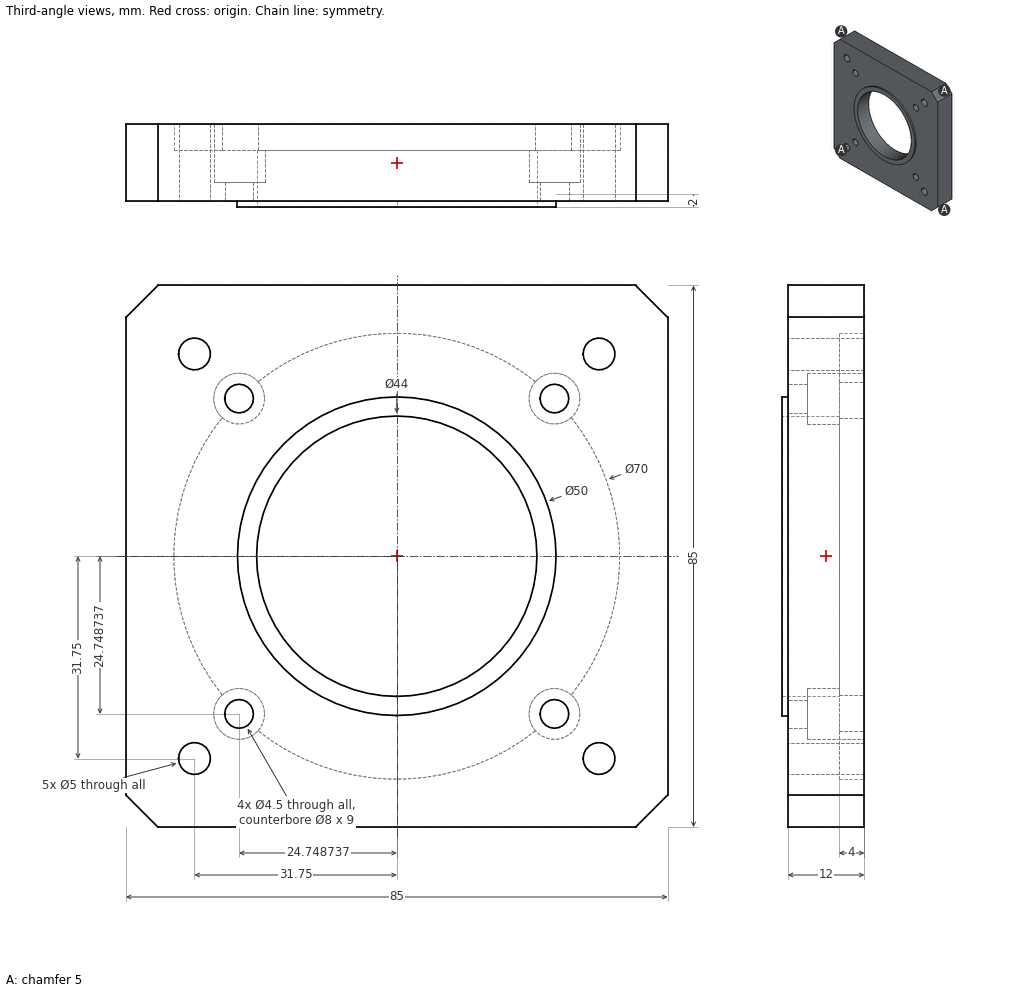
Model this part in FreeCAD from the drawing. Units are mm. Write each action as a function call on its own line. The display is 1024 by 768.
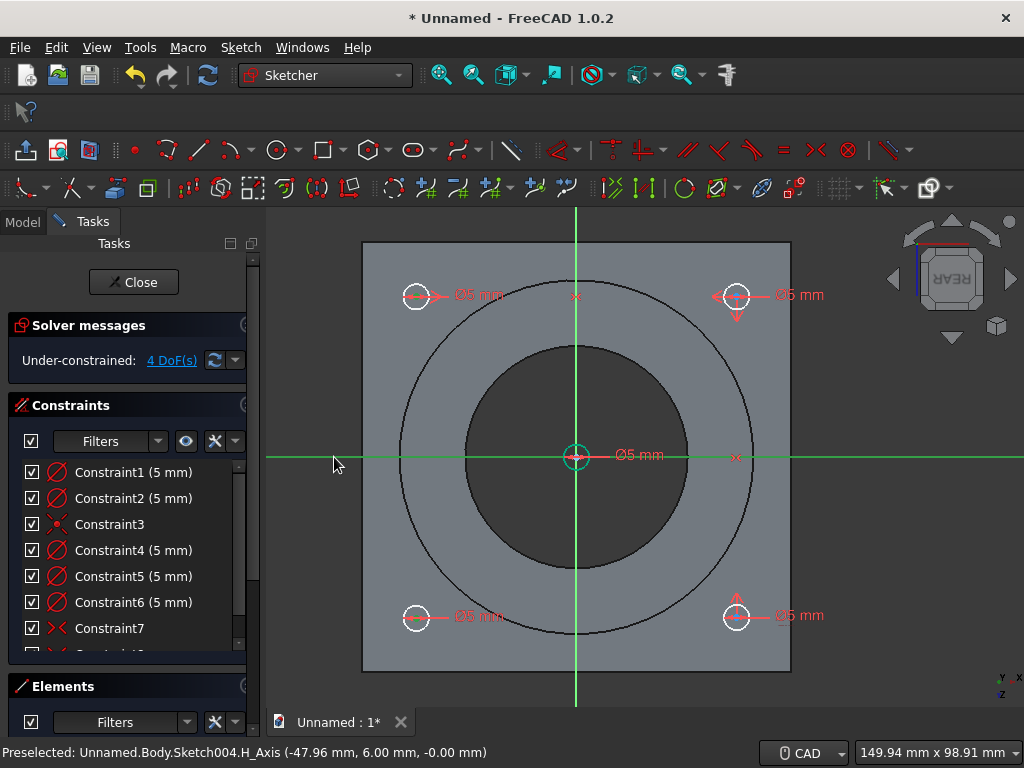
click(816, 150)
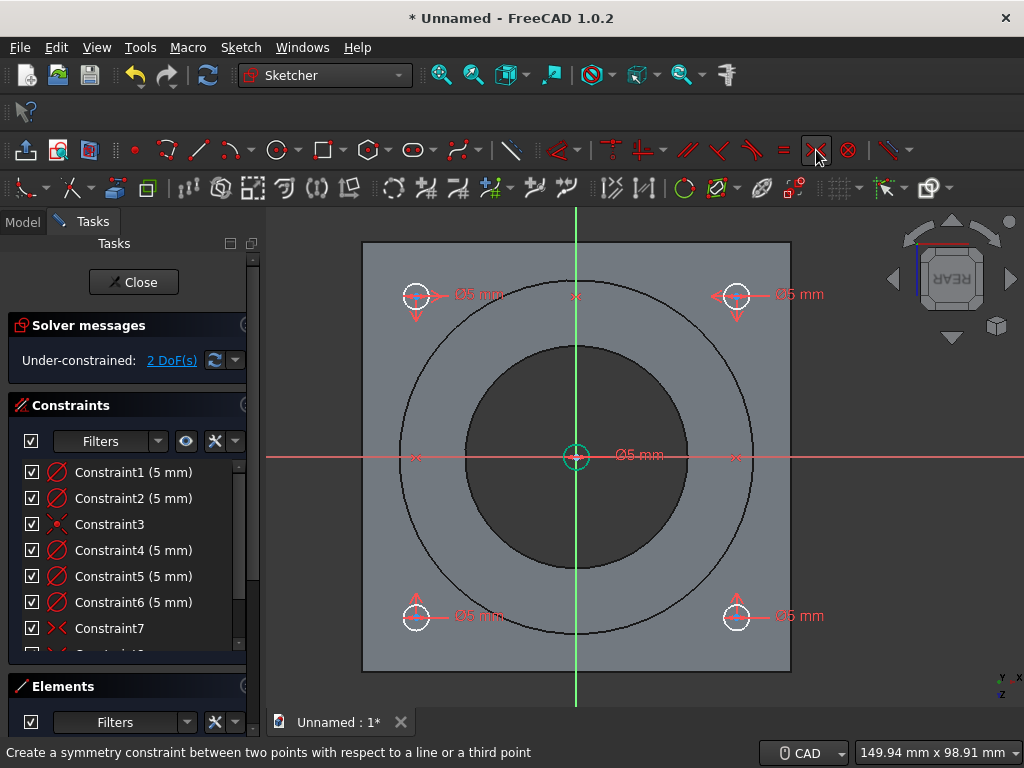
key(d)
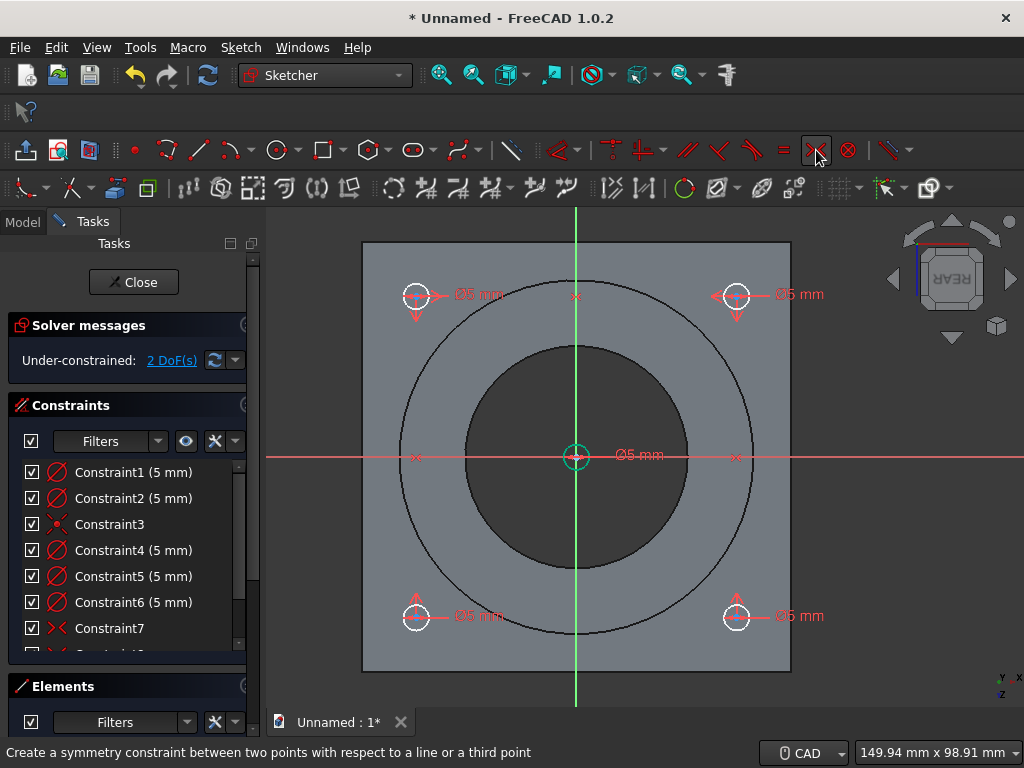
click(416, 296)
click(496, 262)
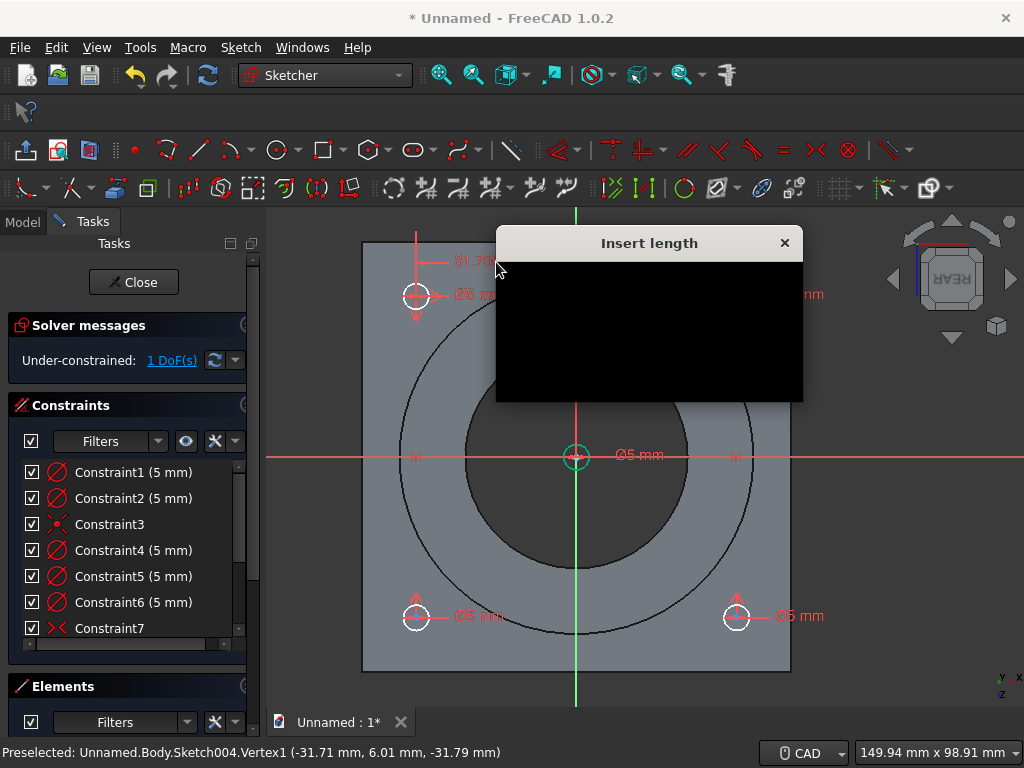
text(31.75)
key(Return)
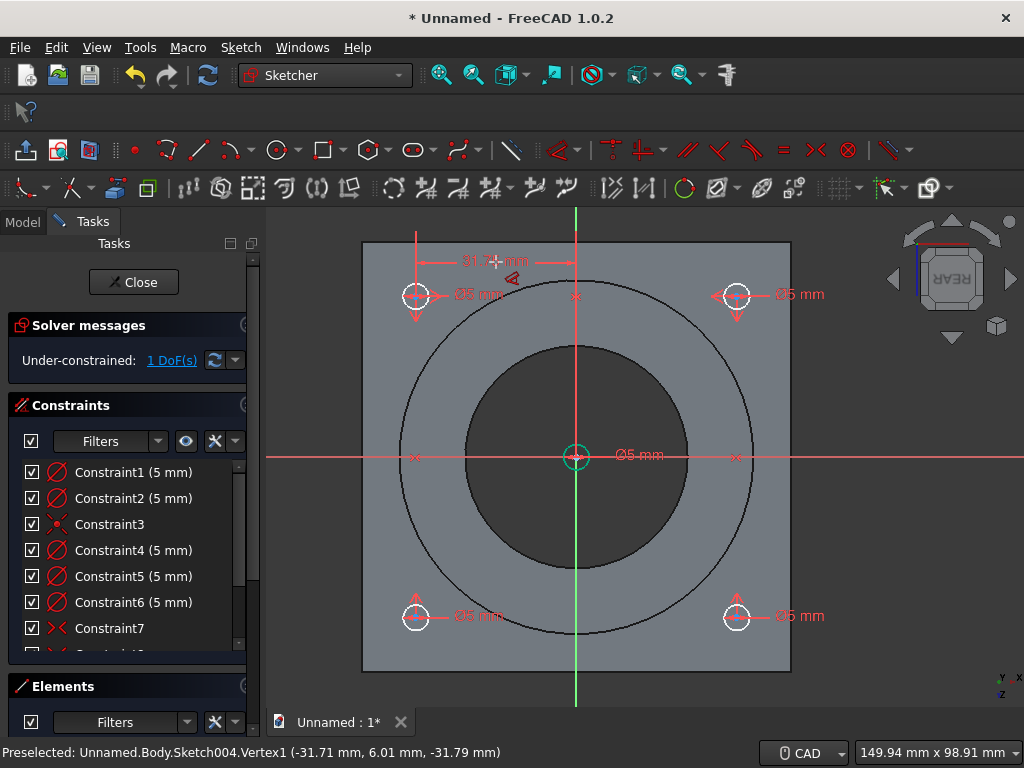
click(416, 296)
click(382, 377)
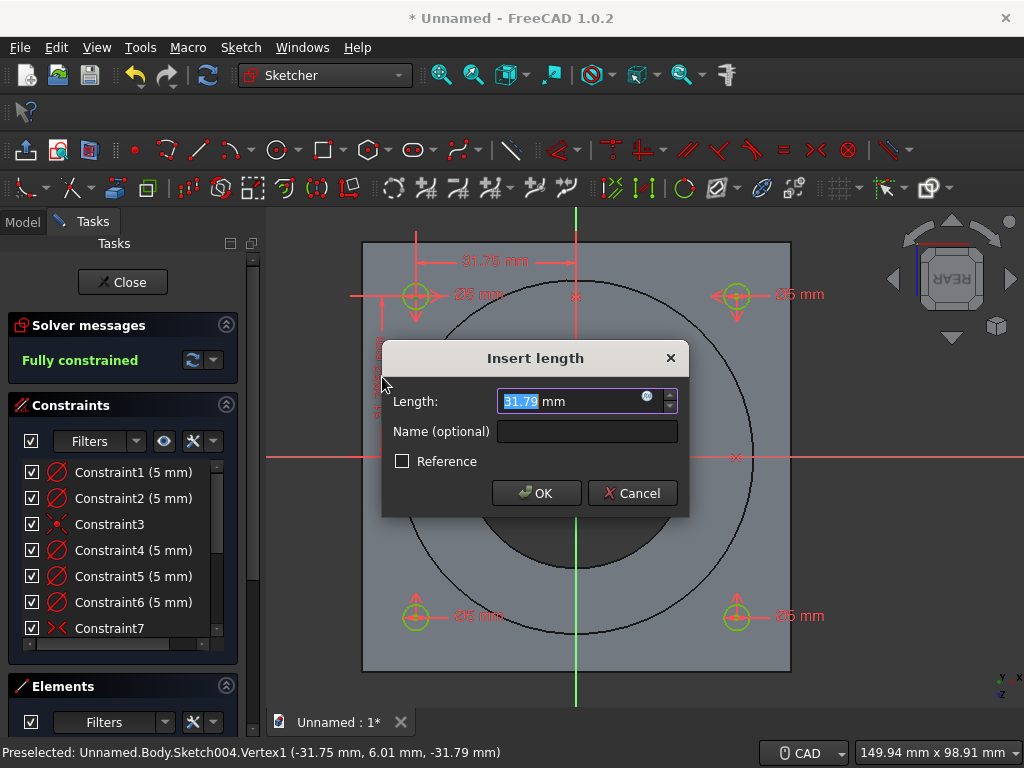
text(31.75)
key(Return)
key(Escape)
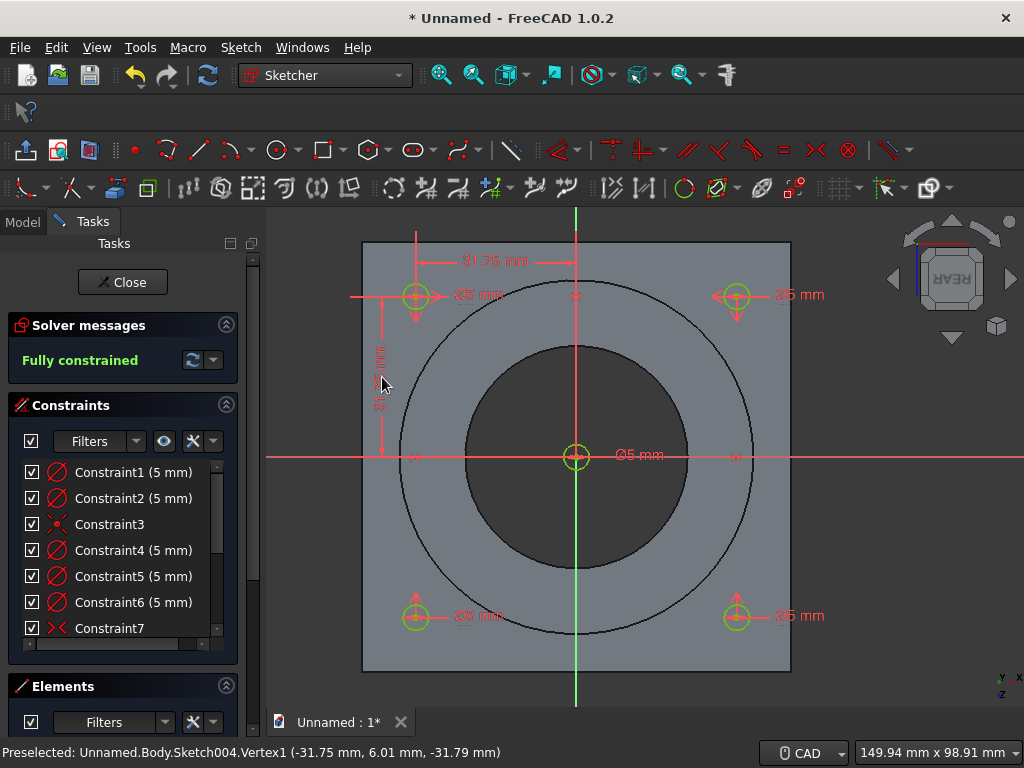
click(123, 282)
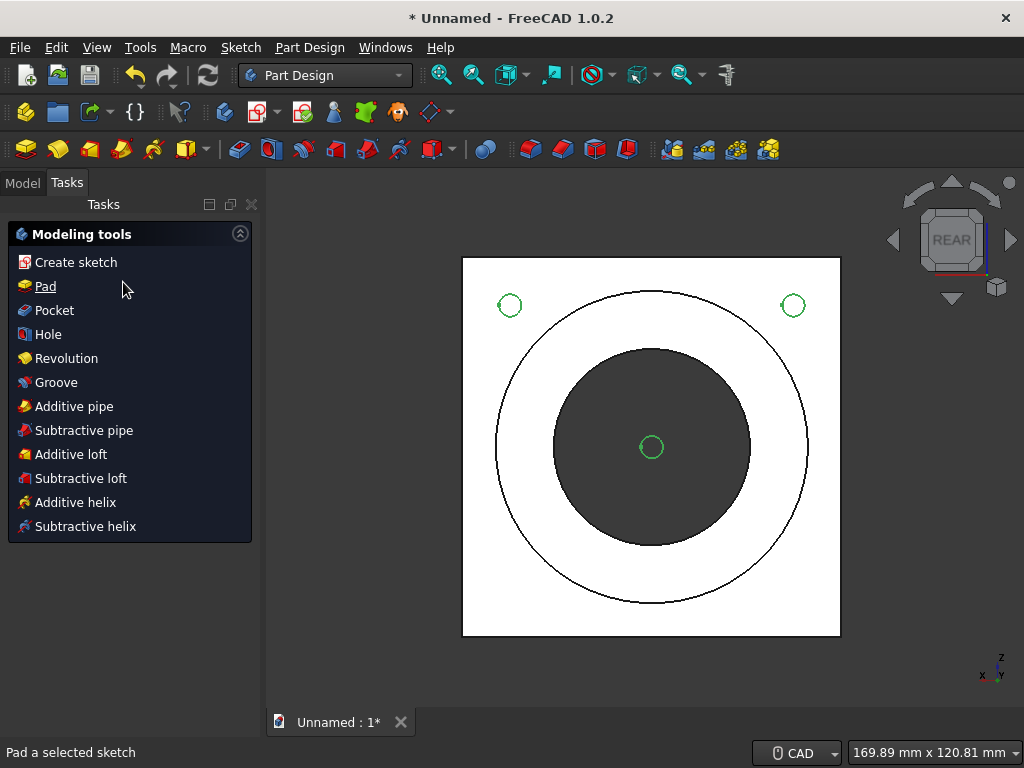
click(272, 150)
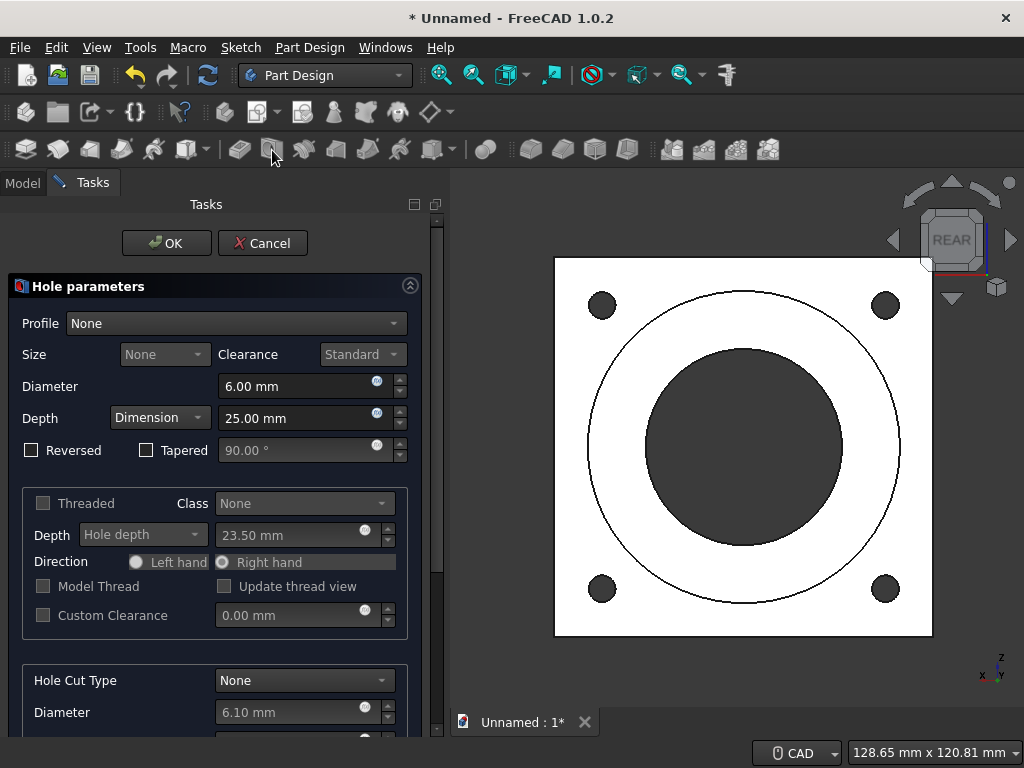
triple_click(305, 386)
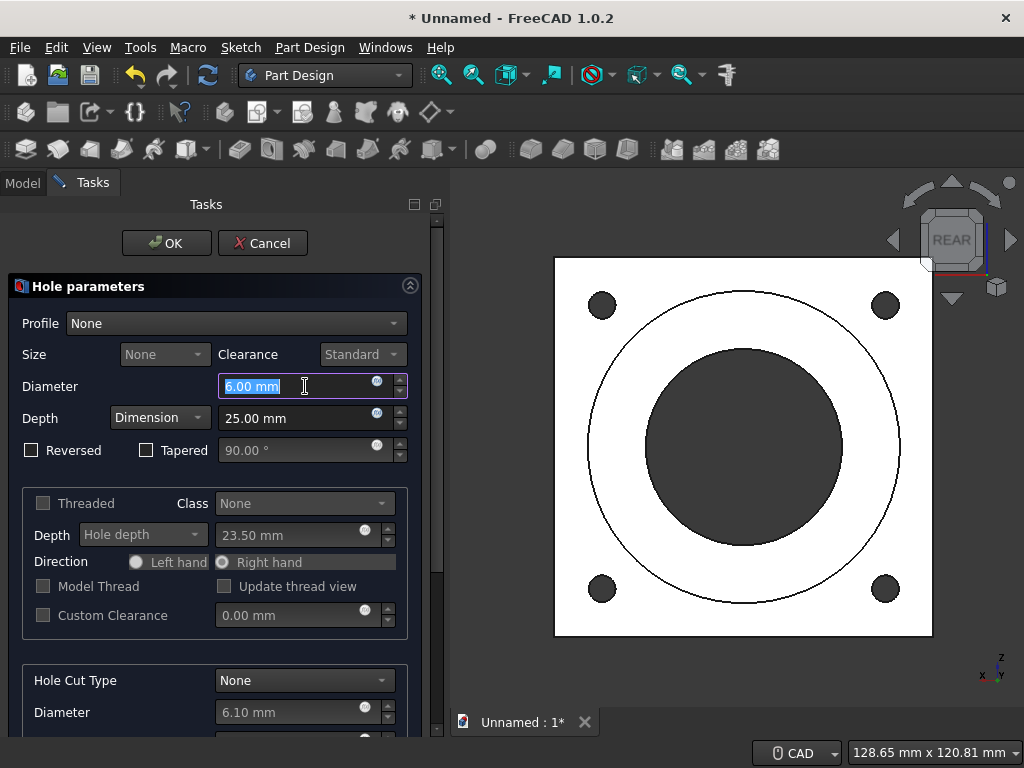
text(5)
key(Tab)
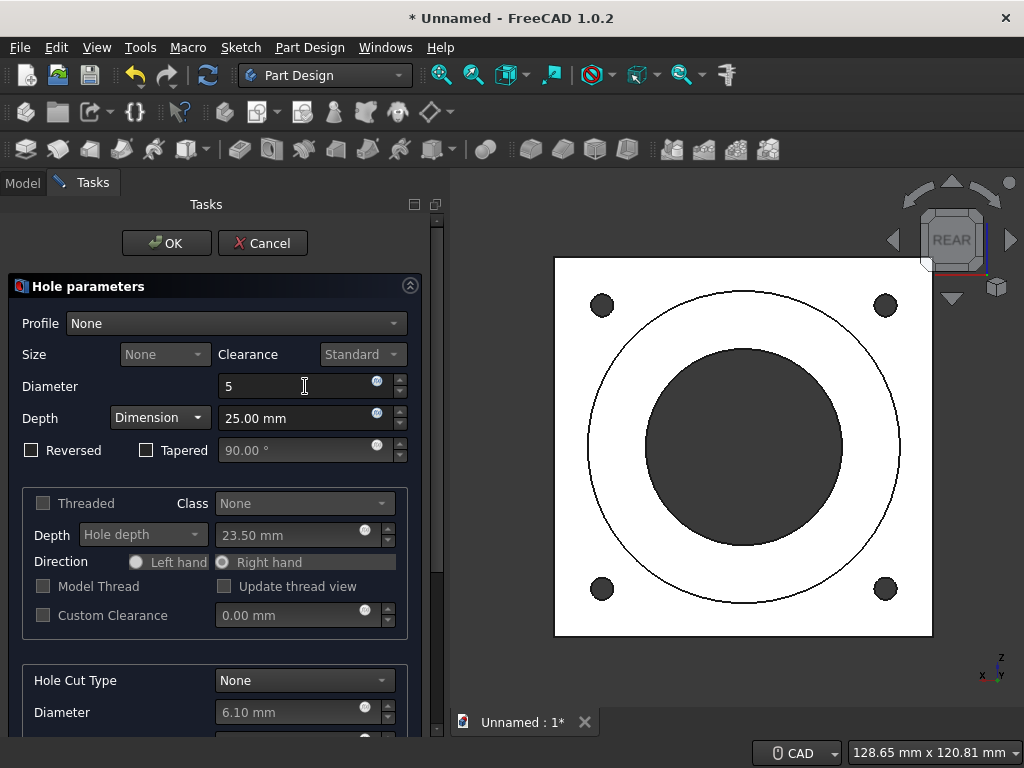
click(161, 418)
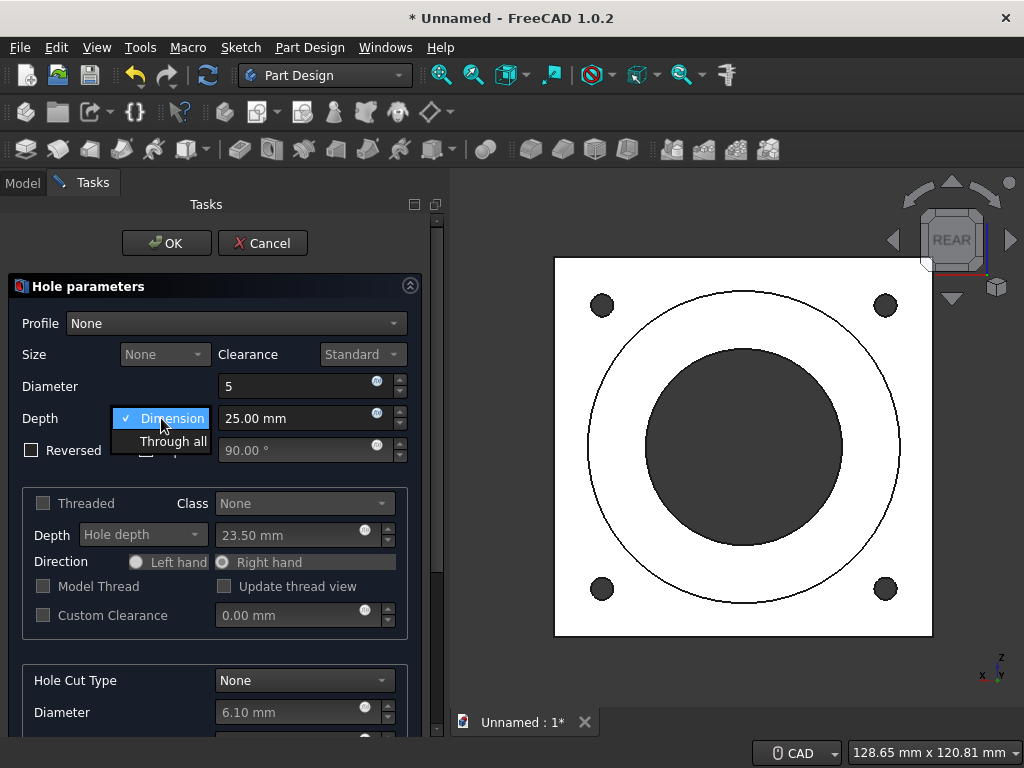
click(160, 442)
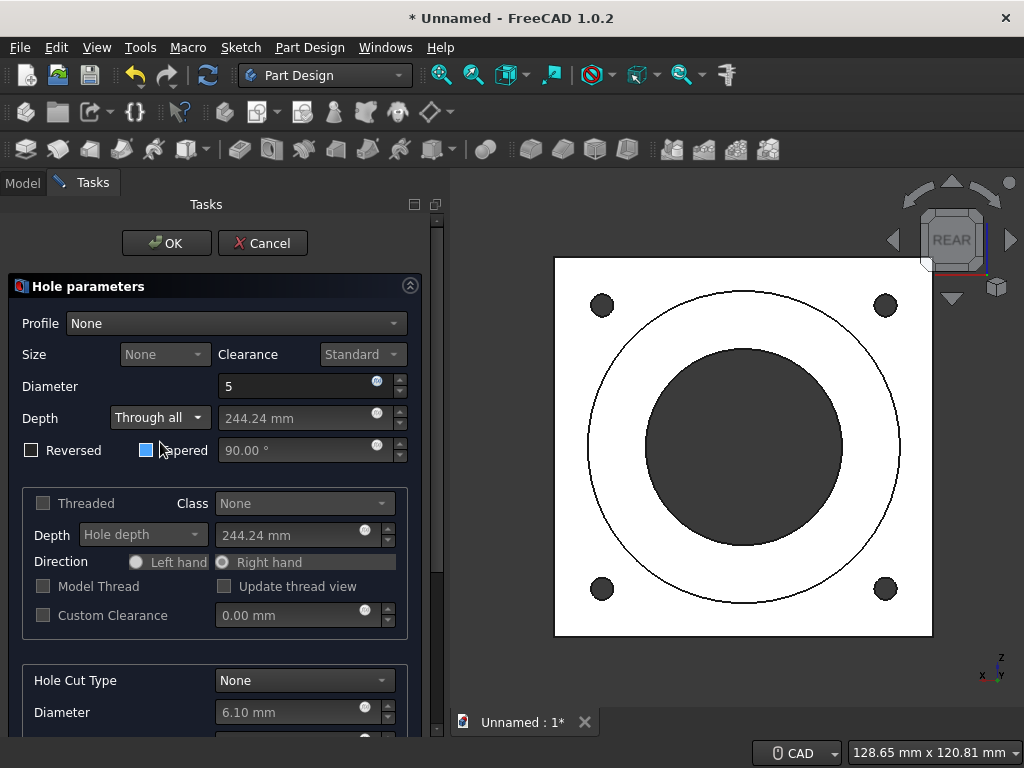
click(167, 243)